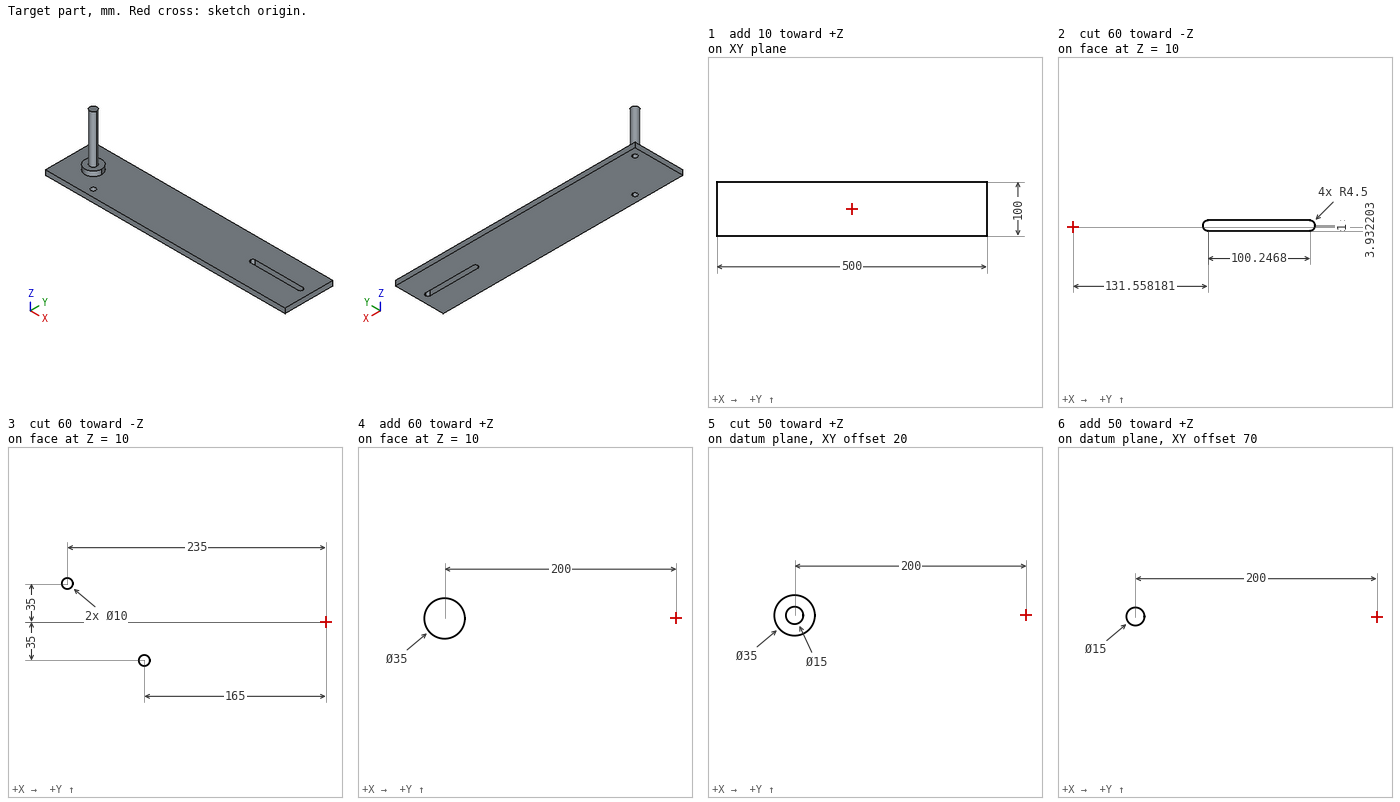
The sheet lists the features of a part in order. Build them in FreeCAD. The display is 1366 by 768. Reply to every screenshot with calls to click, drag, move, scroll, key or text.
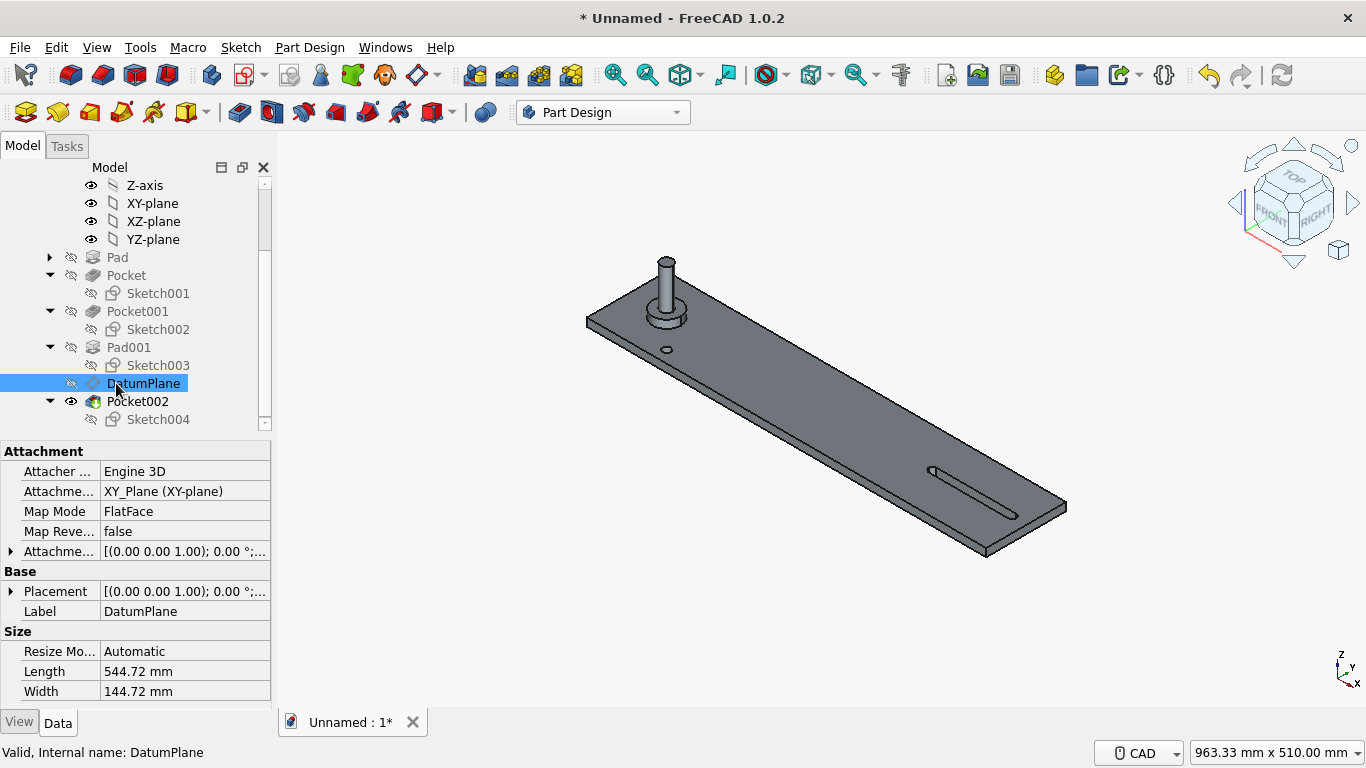
key(2)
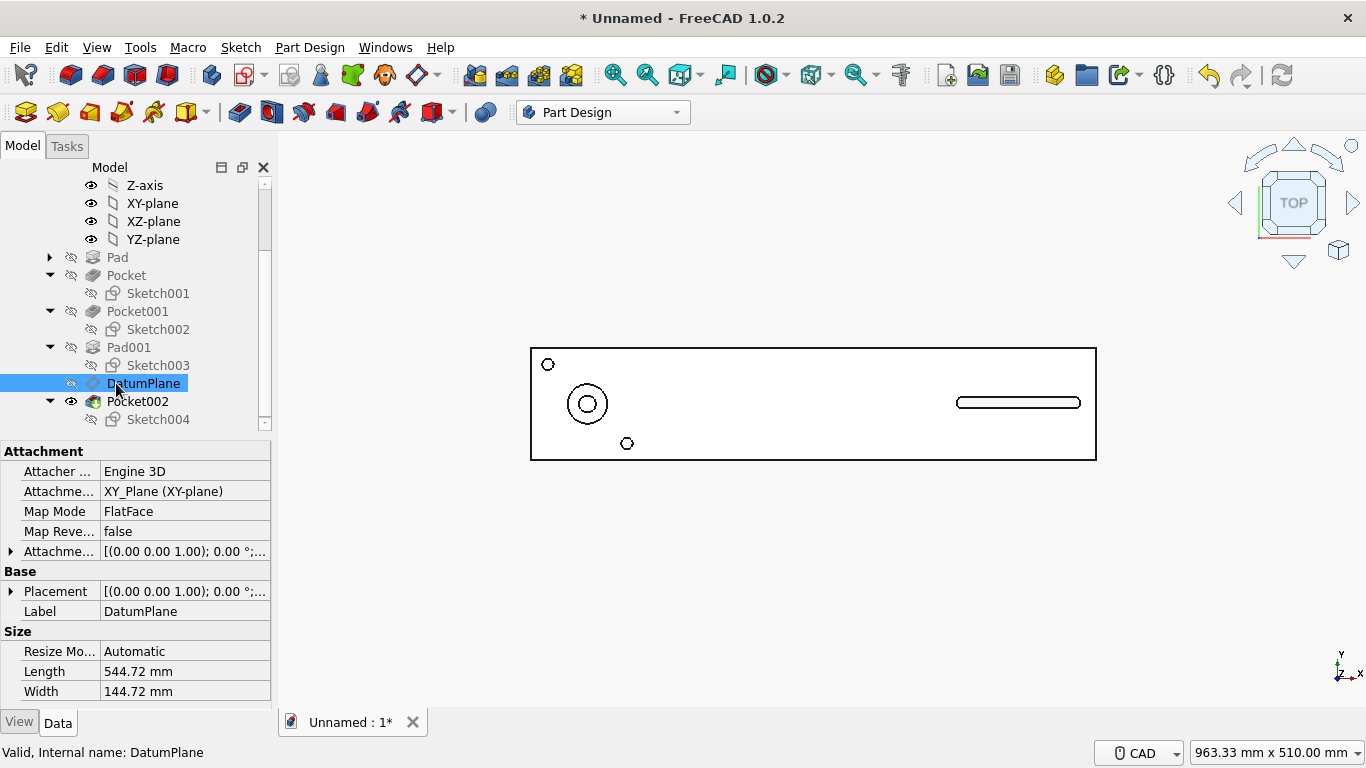
key(1)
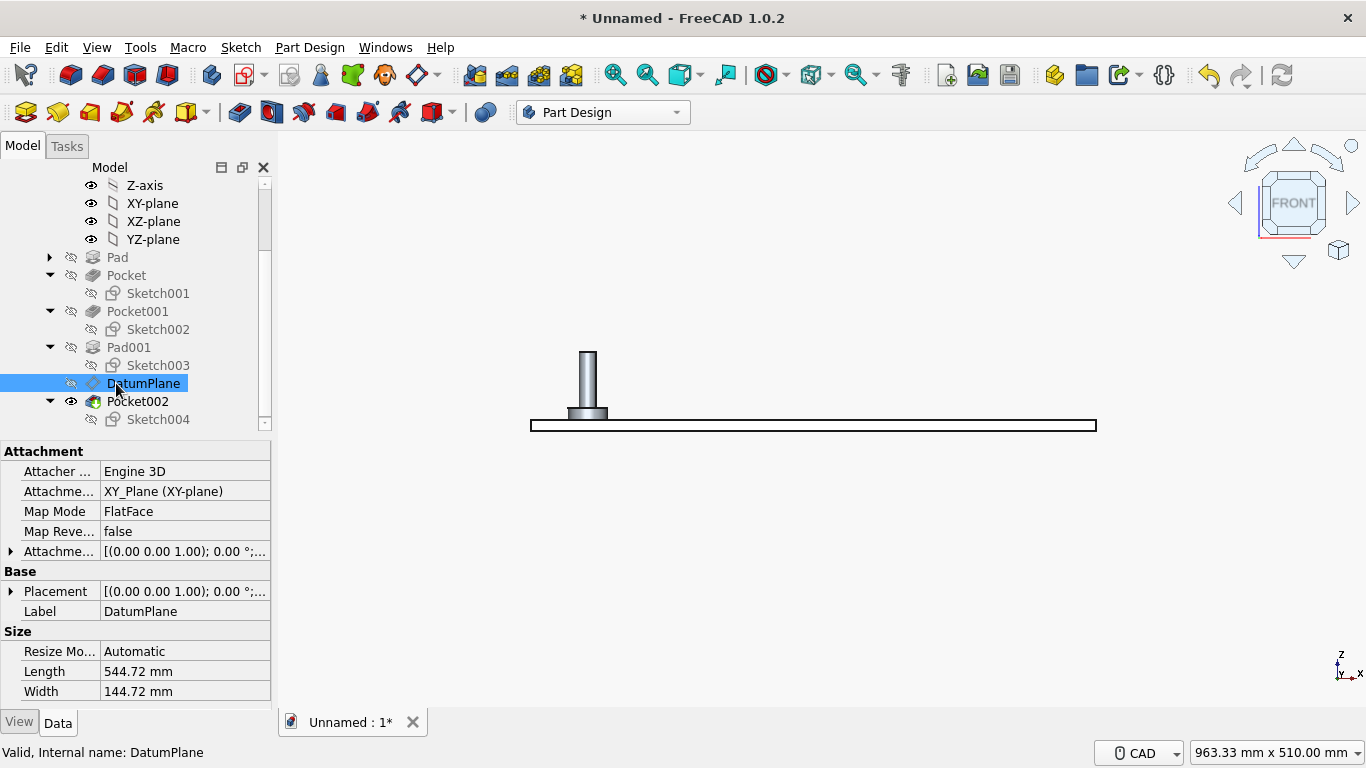
scroll(160, 307, down, 3)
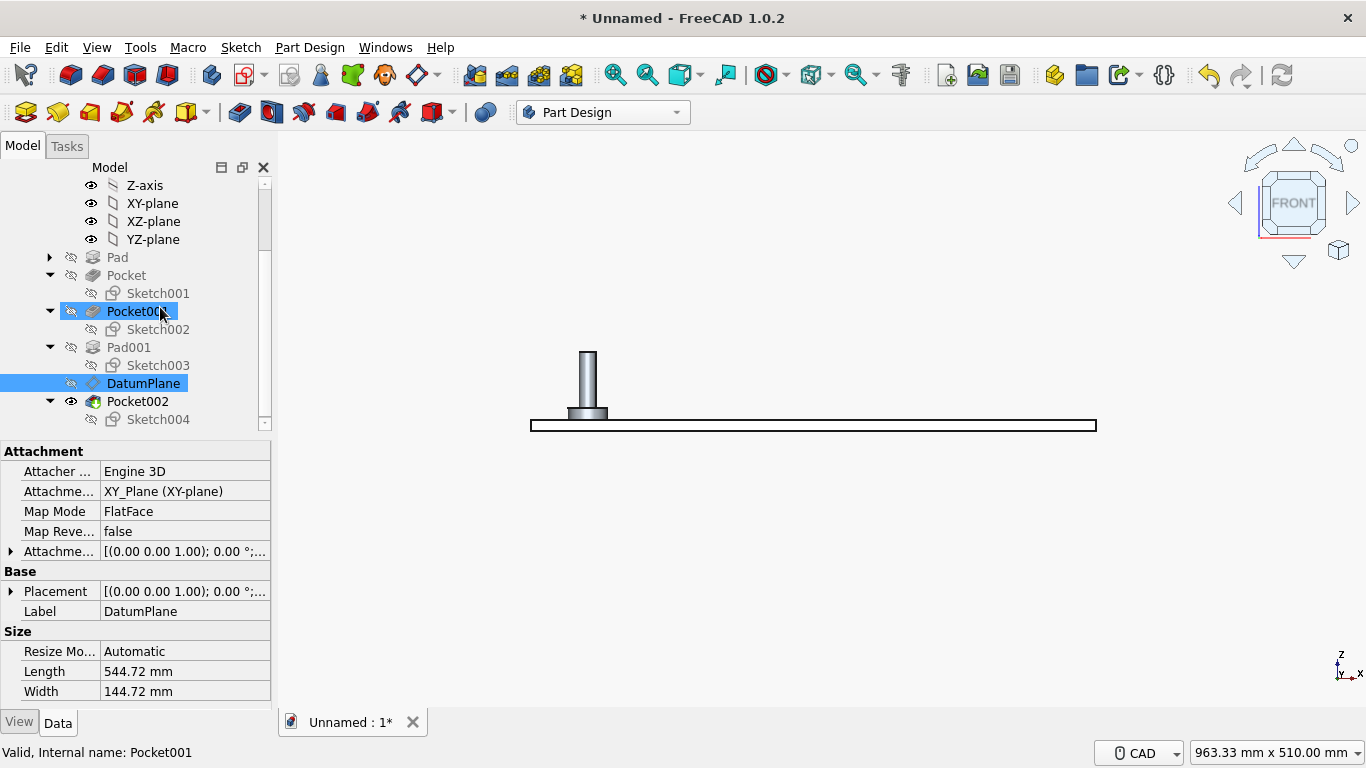
scroll(160, 307, up, 15)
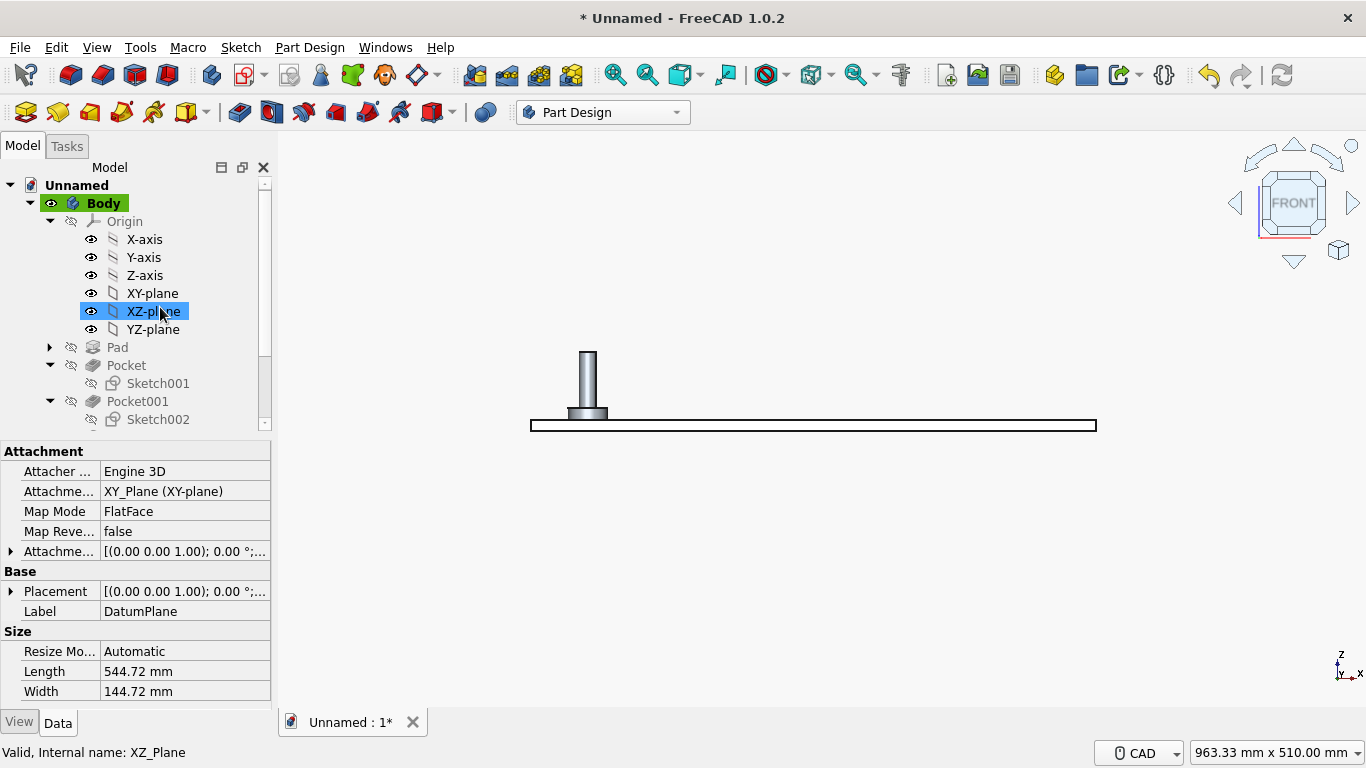
click(136, 293)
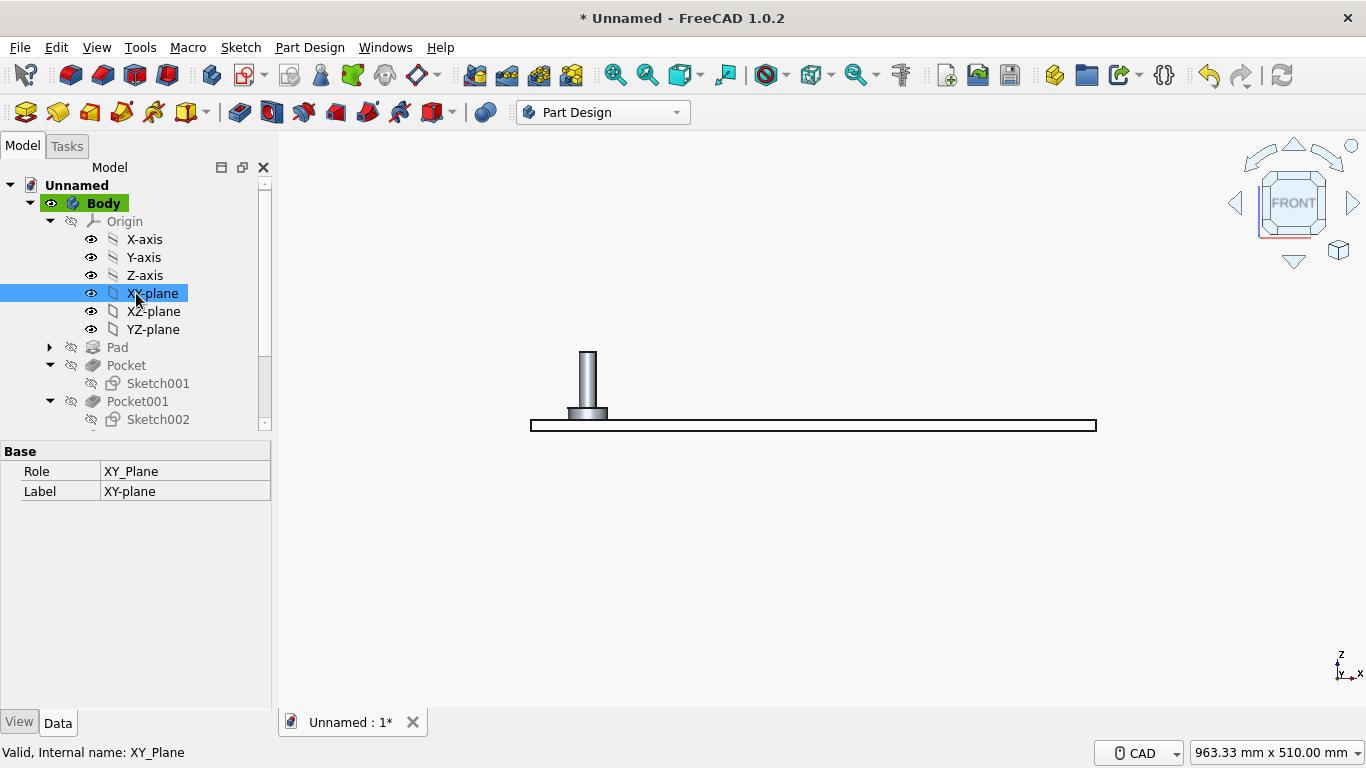
click(418, 76)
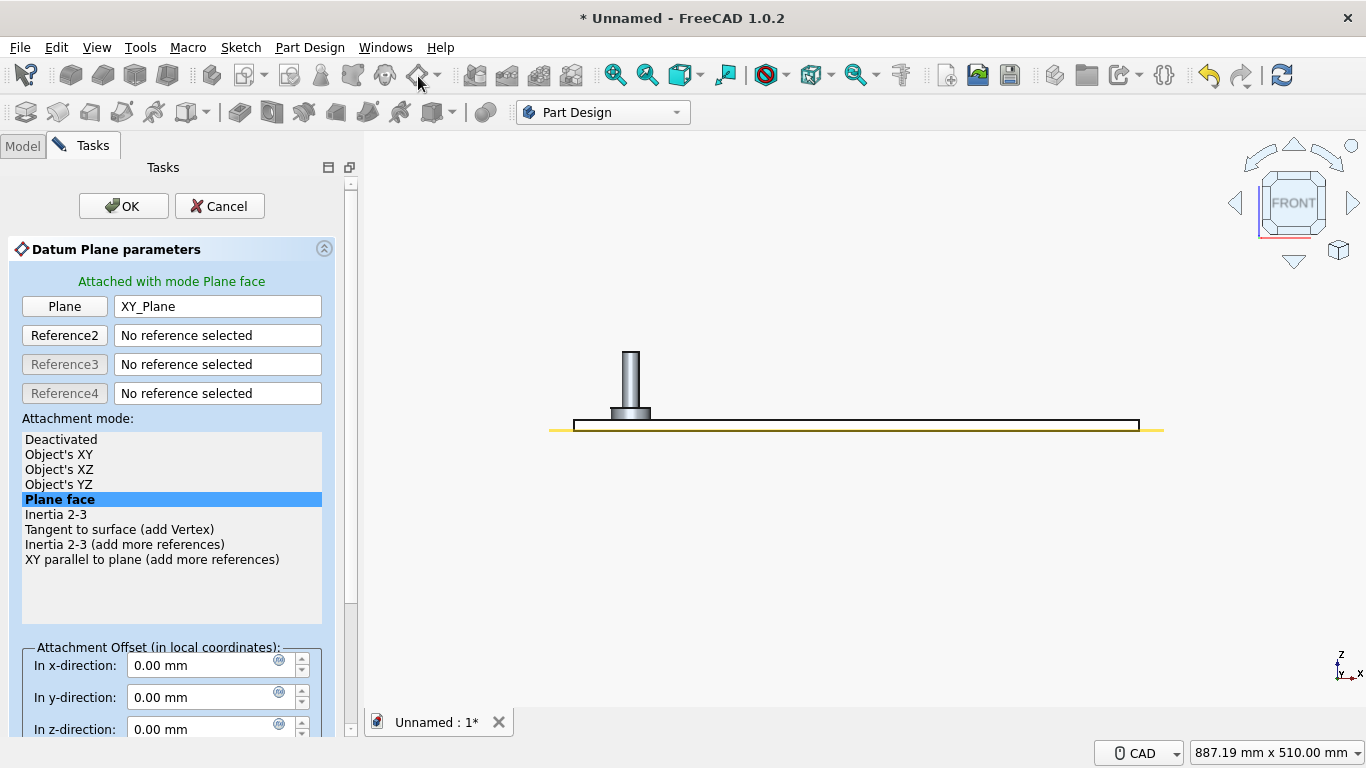
scroll(351, 456, down, 2)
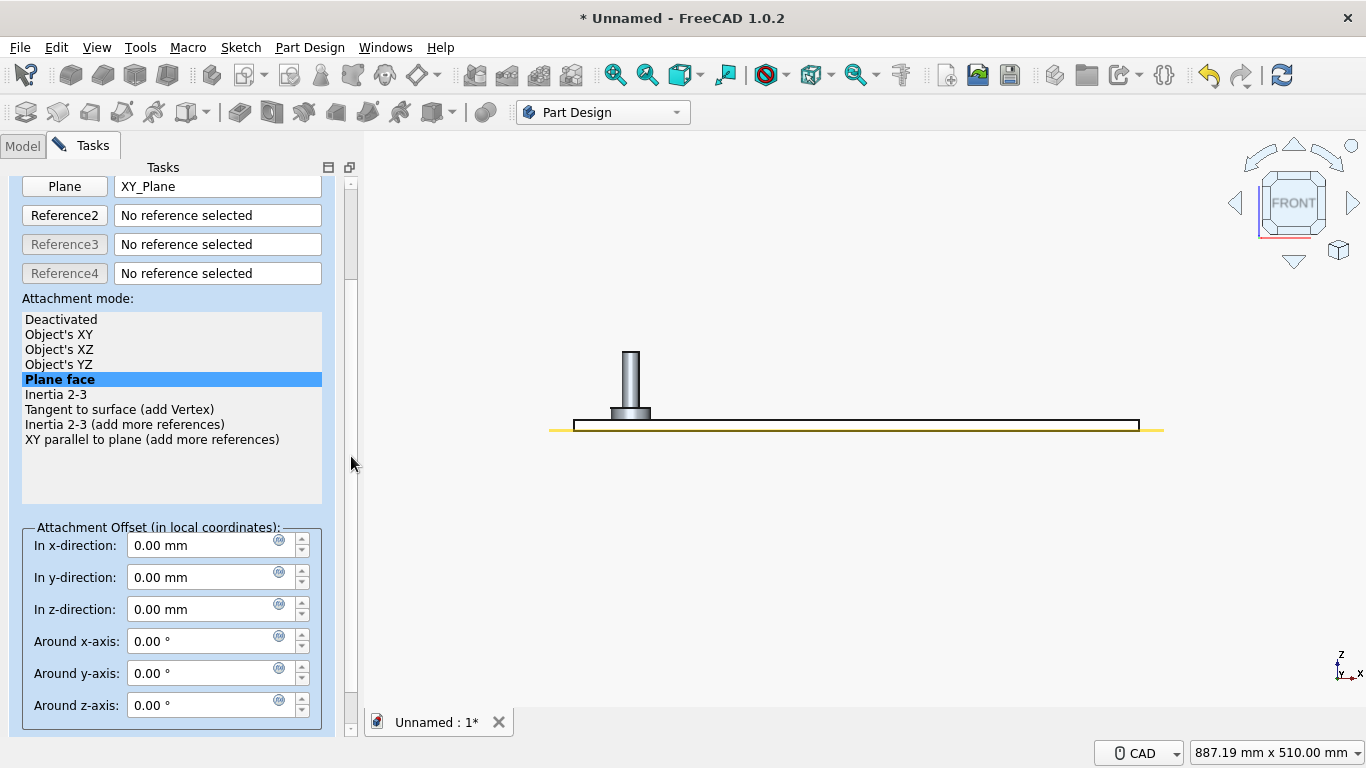
triple_click(210, 609)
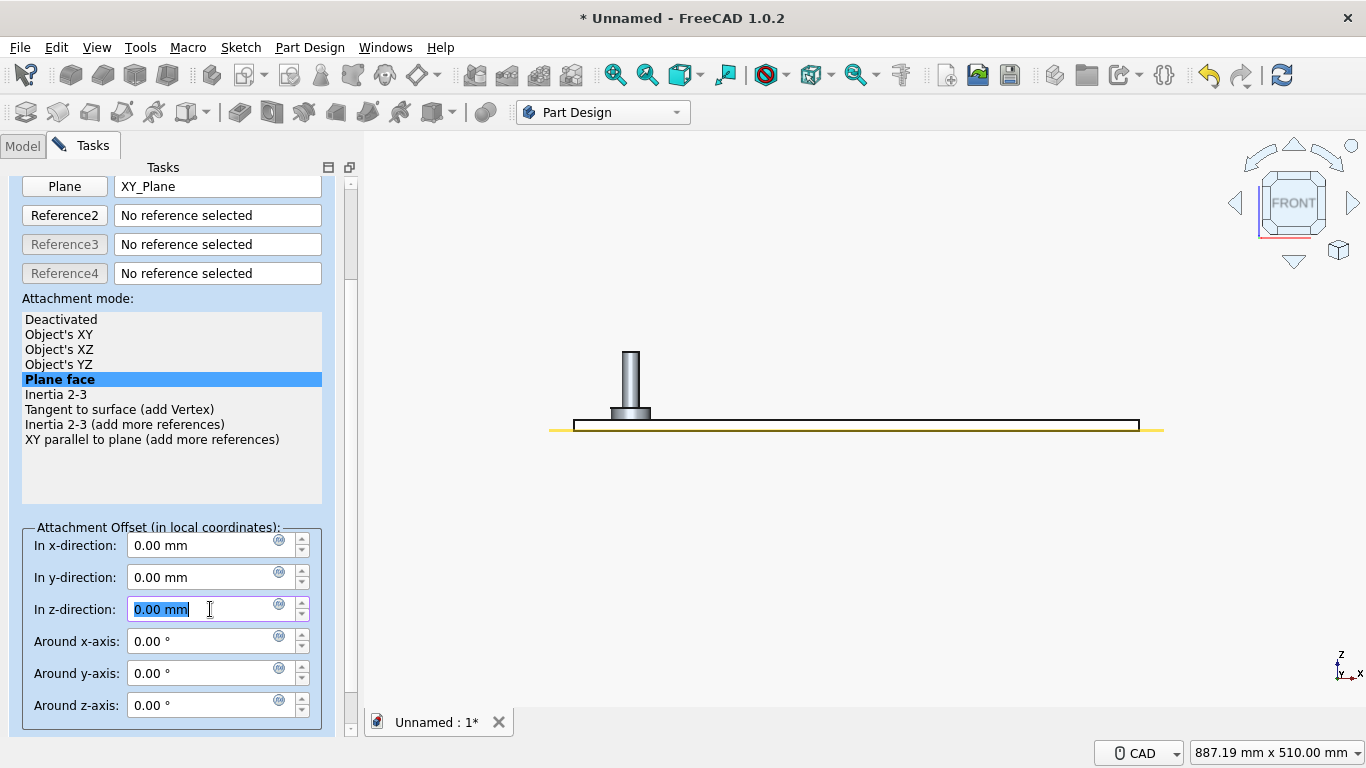
text(70)
key(Tab)